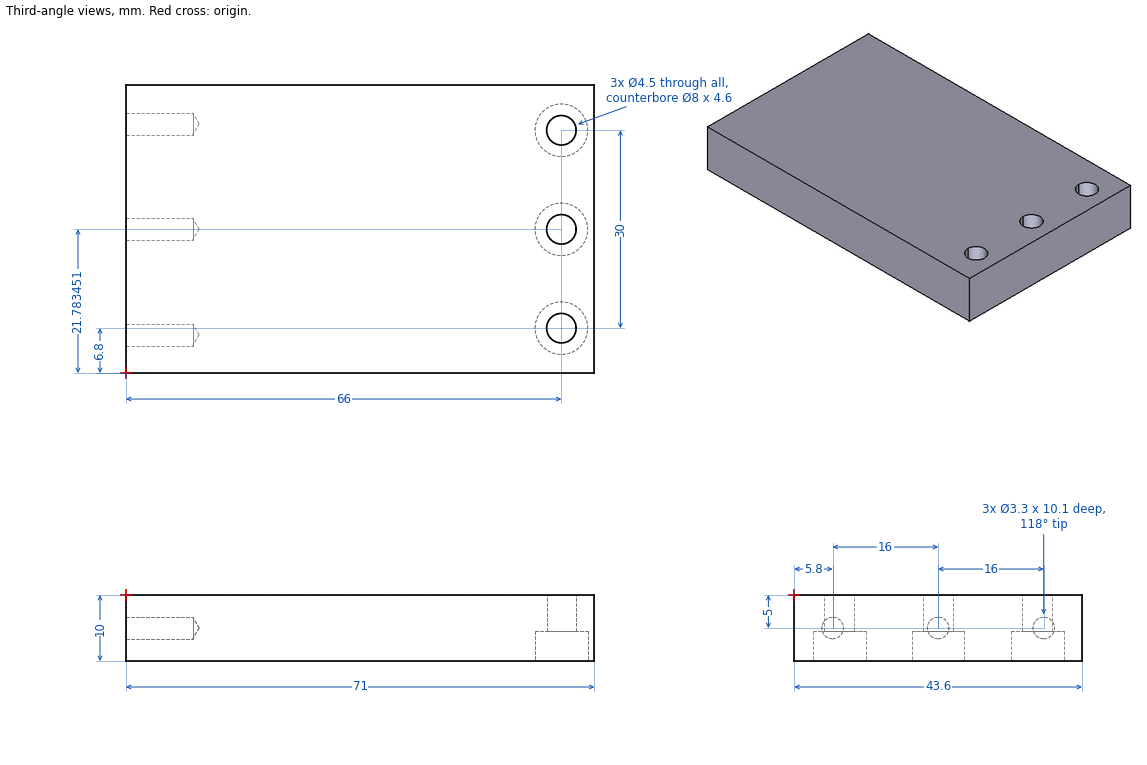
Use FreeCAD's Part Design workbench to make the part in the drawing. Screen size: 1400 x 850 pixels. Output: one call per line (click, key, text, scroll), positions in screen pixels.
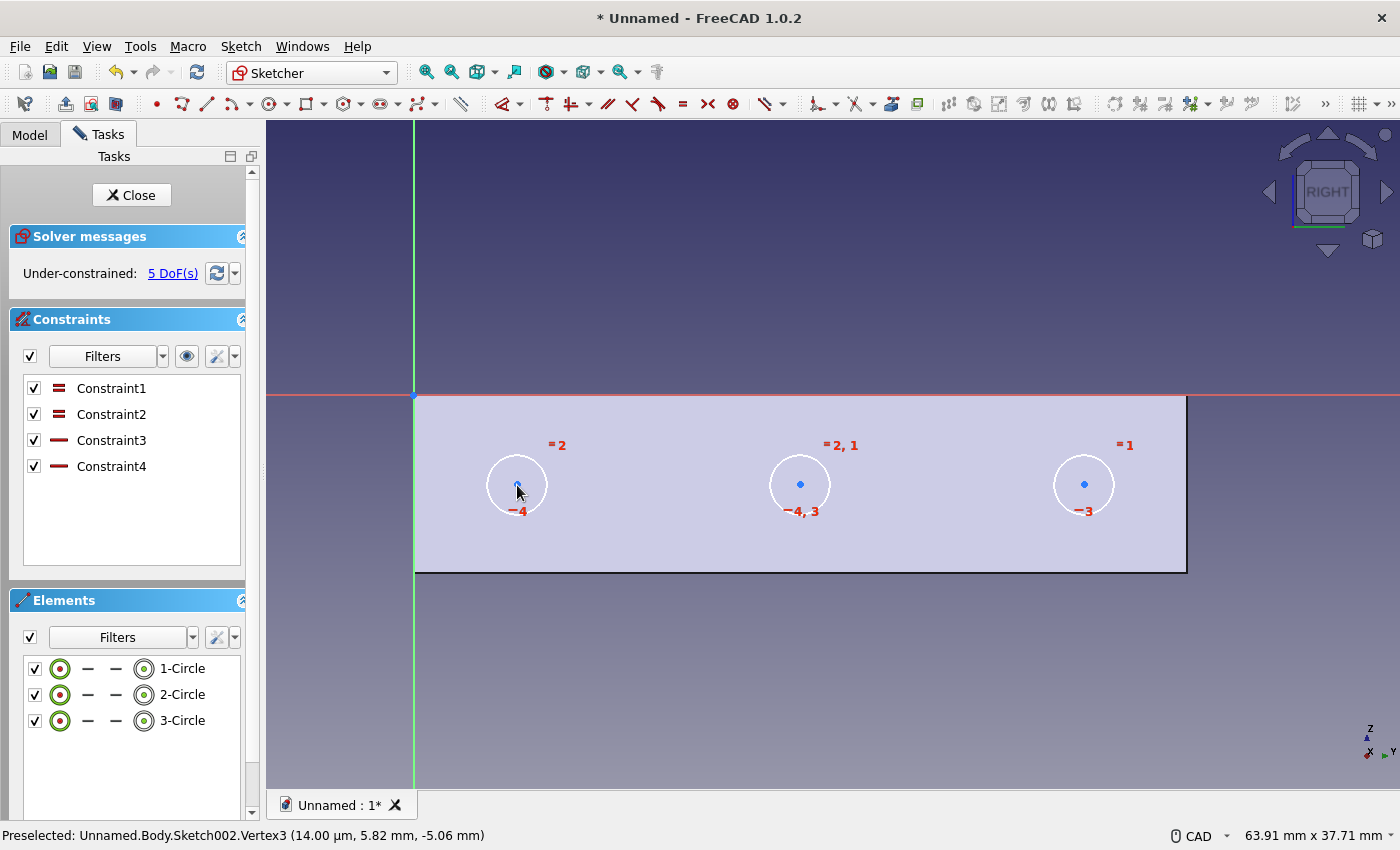
key(d)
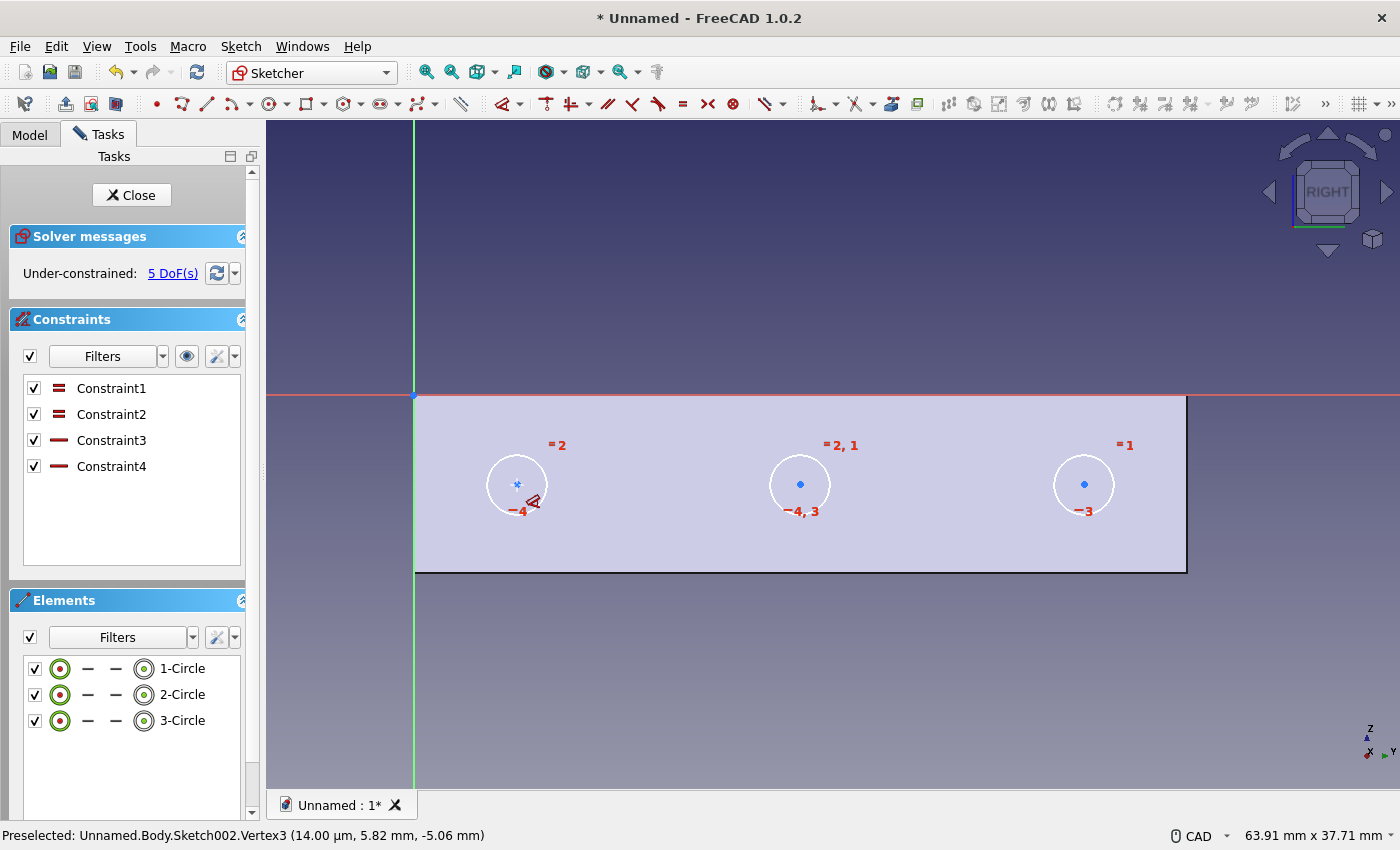
click(1105, 464)
click(1128, 441)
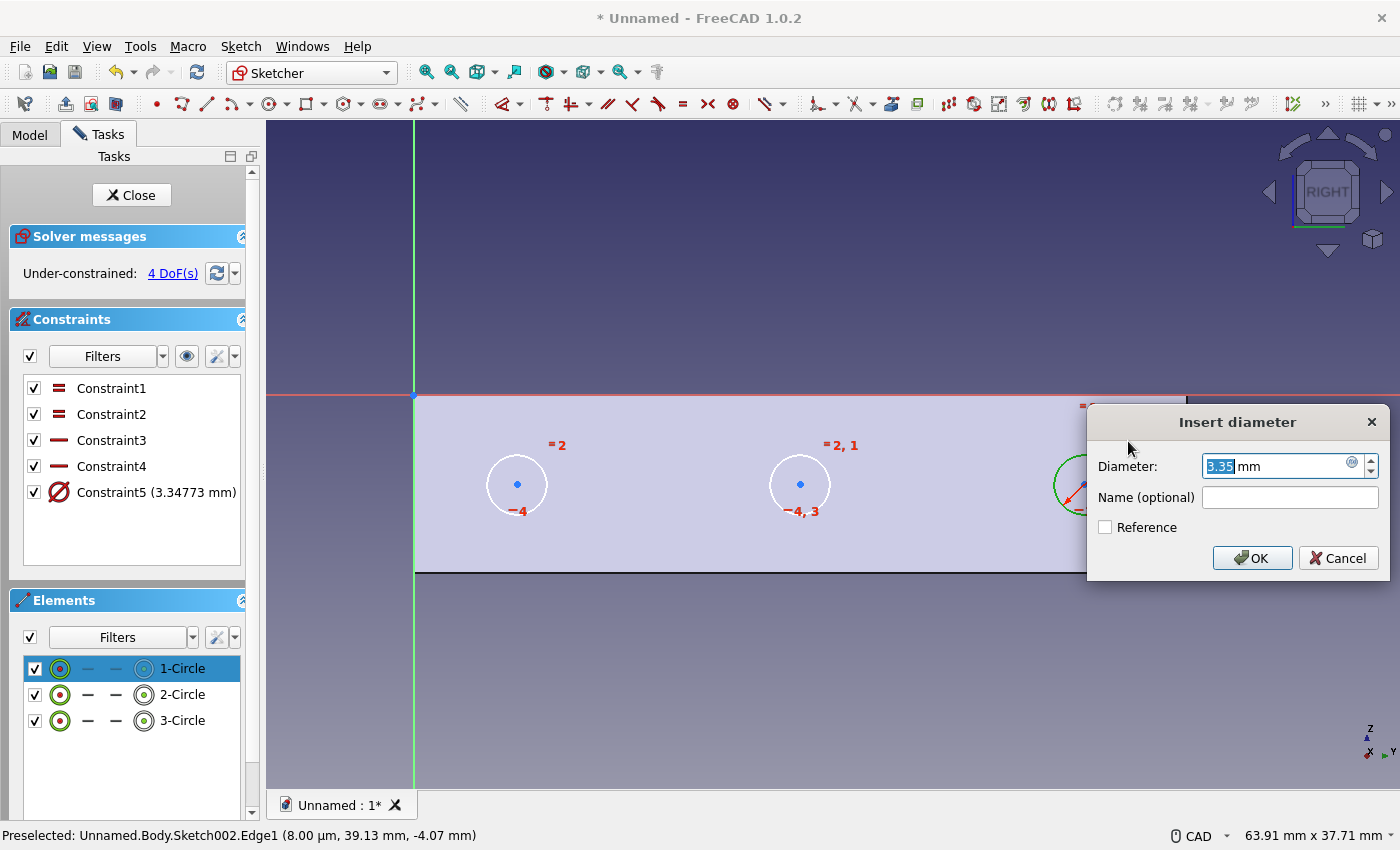
text(3.3)
key(Return)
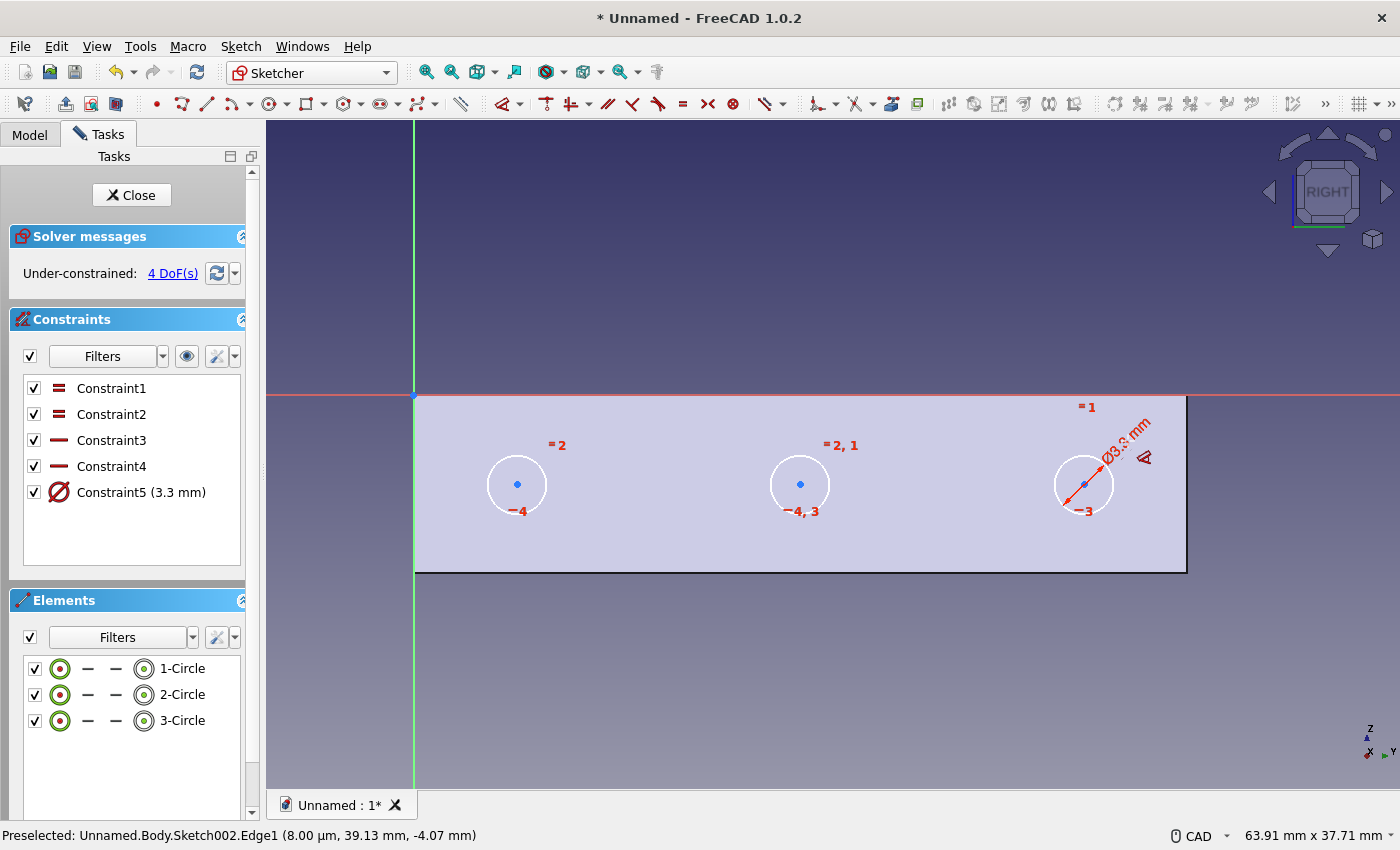
click(1084, 485)
click(380, 440)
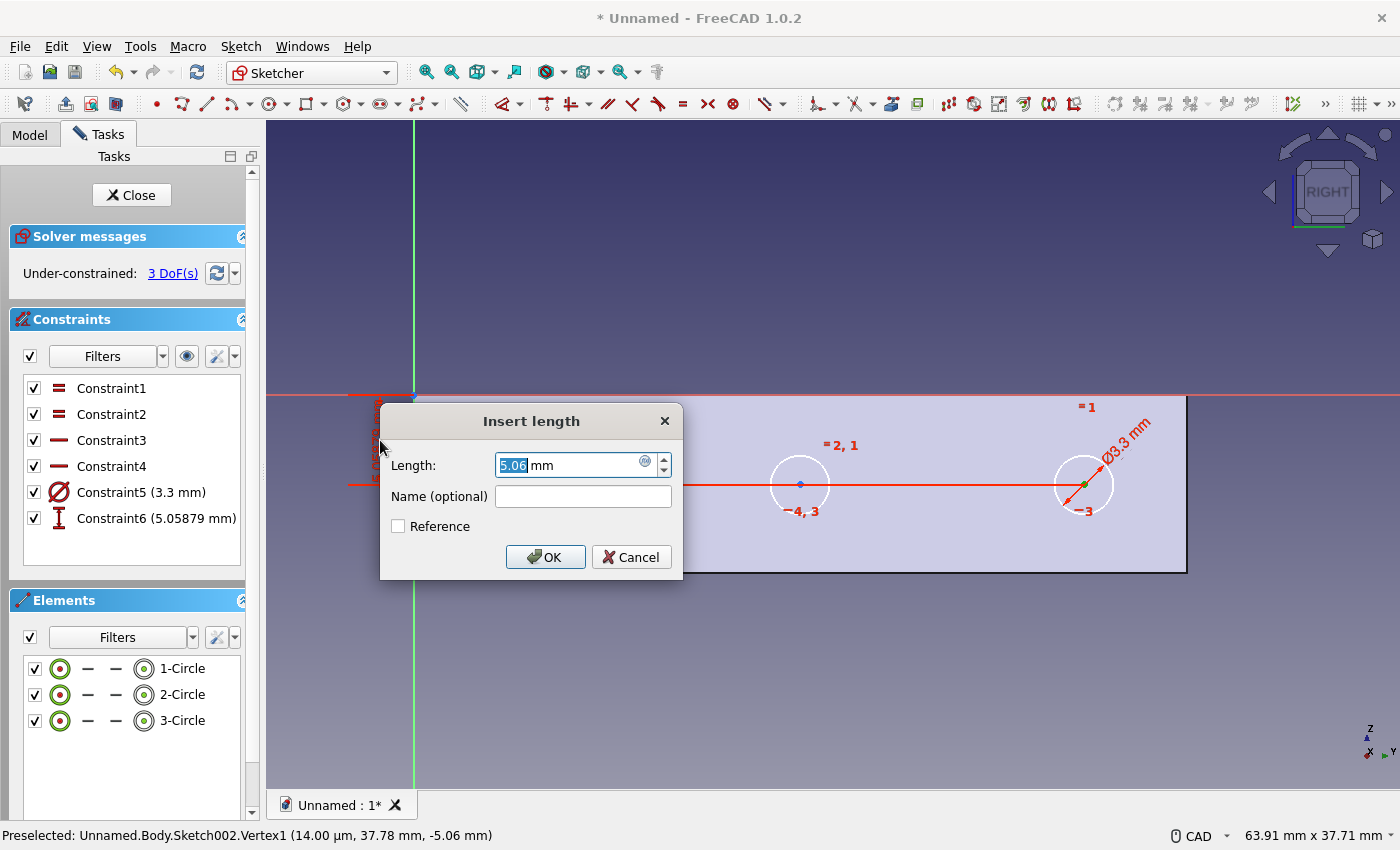
text(5)
key(Return)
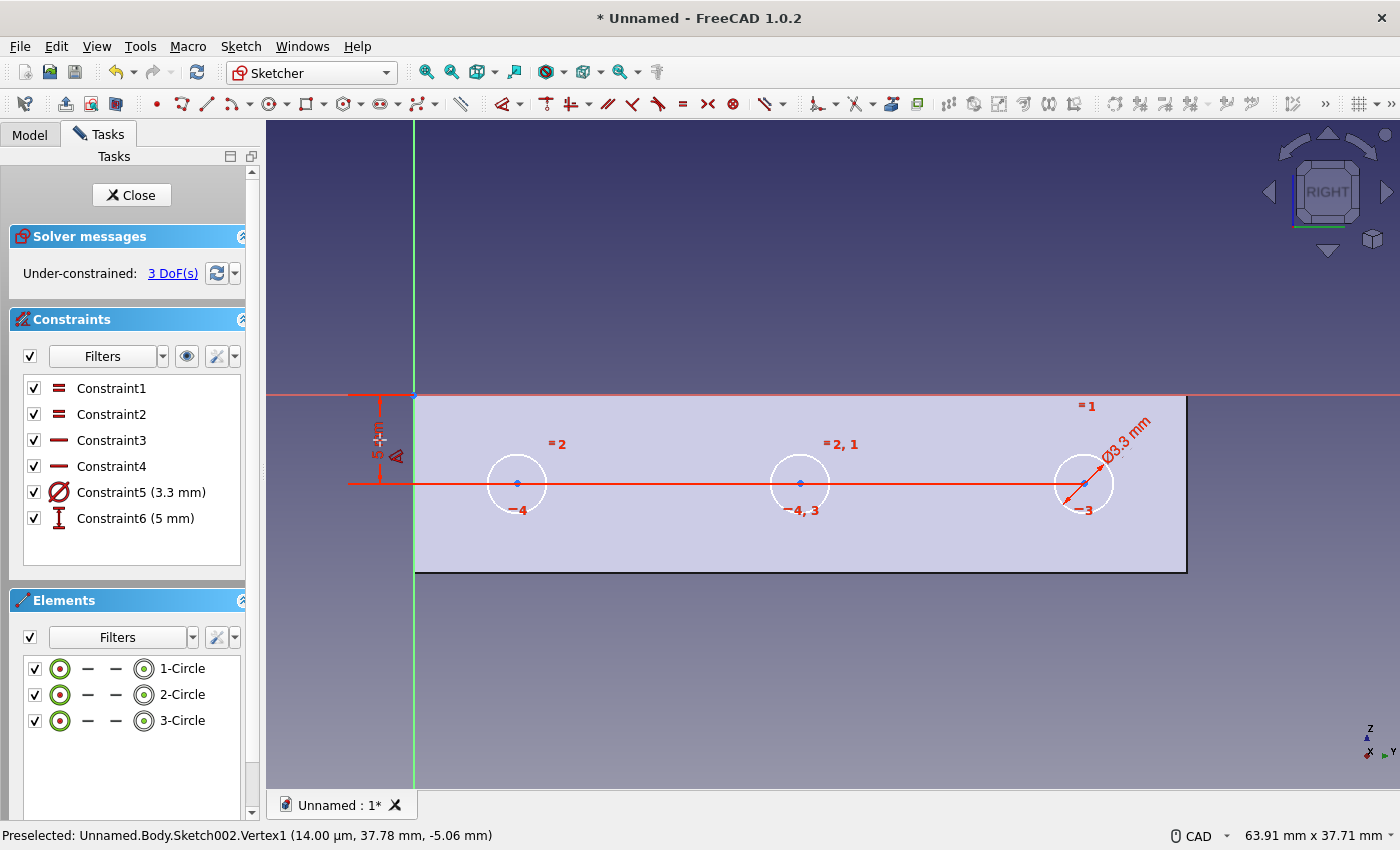
click(517, 484)
click(465, 361)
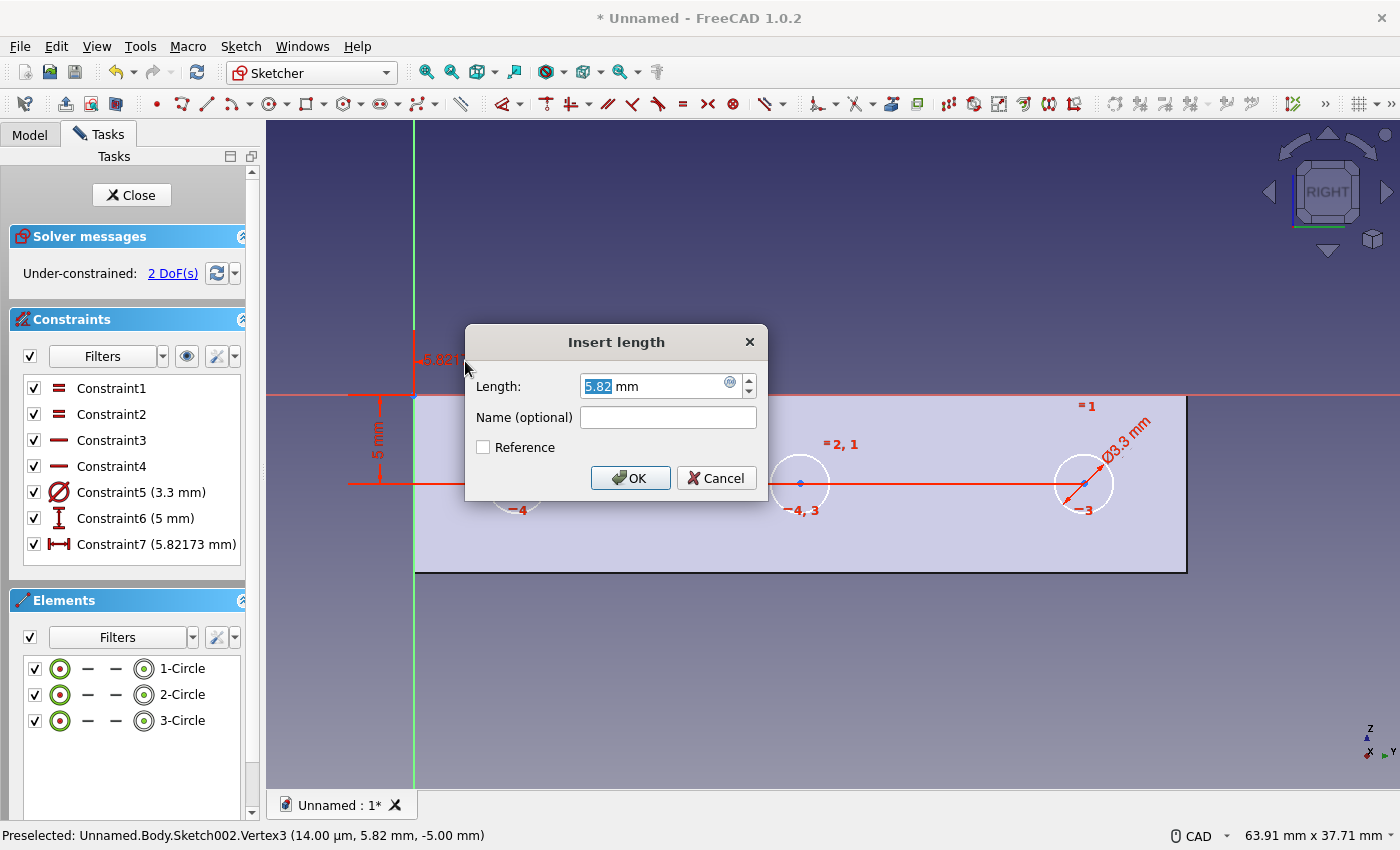
text(5.8)
key(Return)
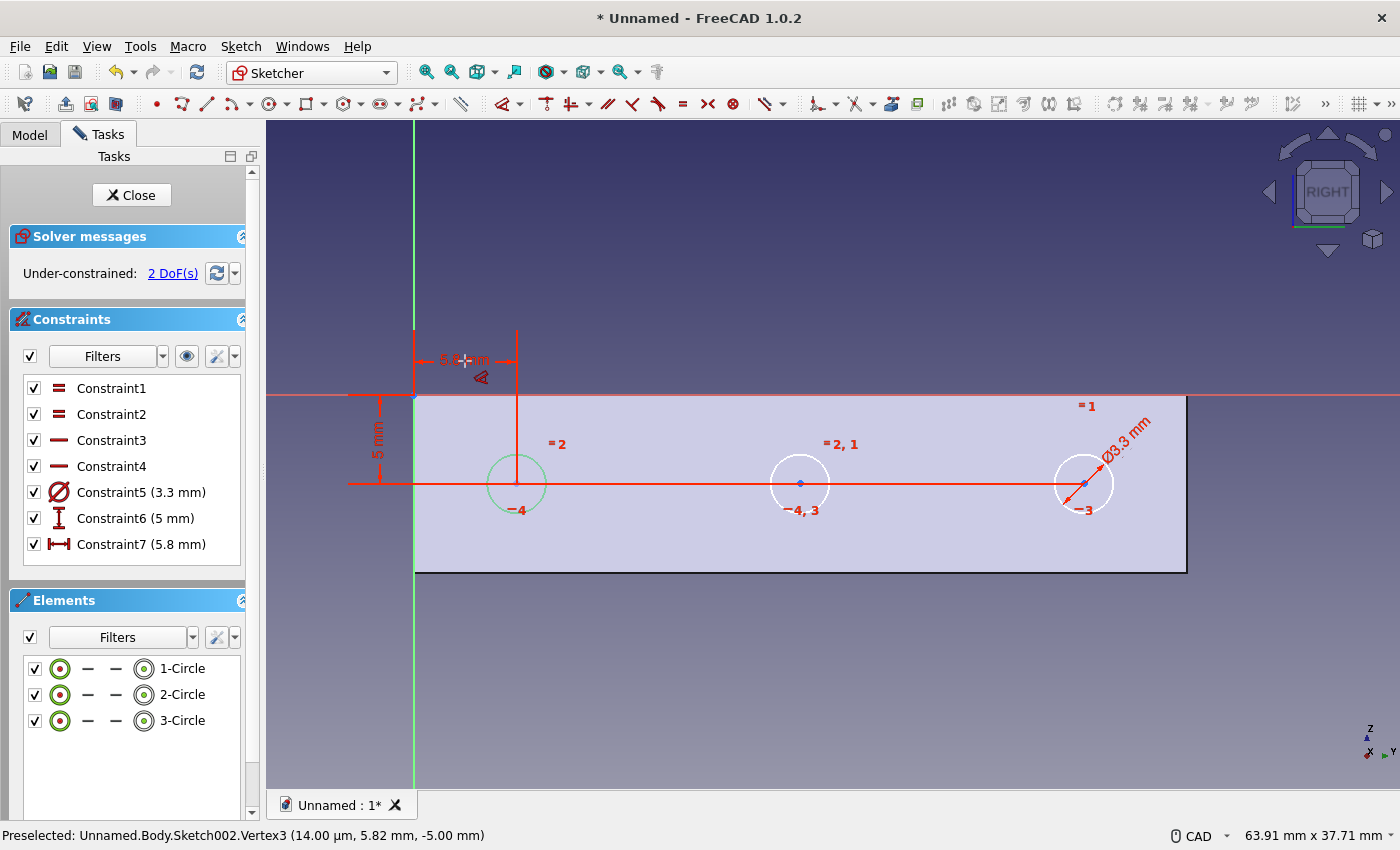
click(1084, 484)